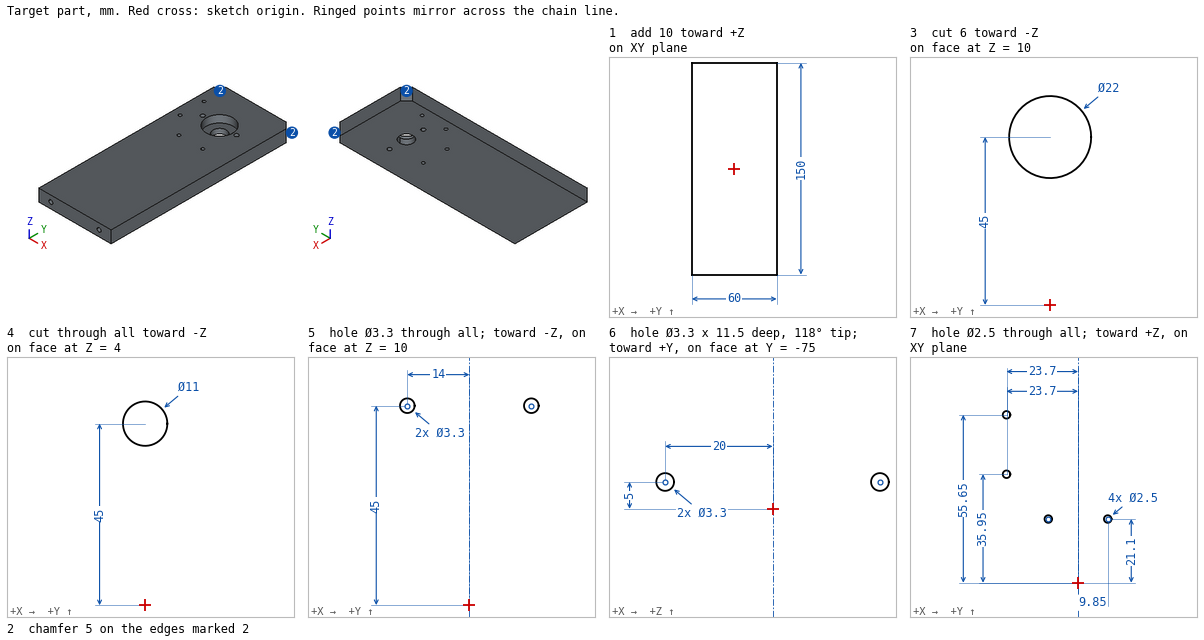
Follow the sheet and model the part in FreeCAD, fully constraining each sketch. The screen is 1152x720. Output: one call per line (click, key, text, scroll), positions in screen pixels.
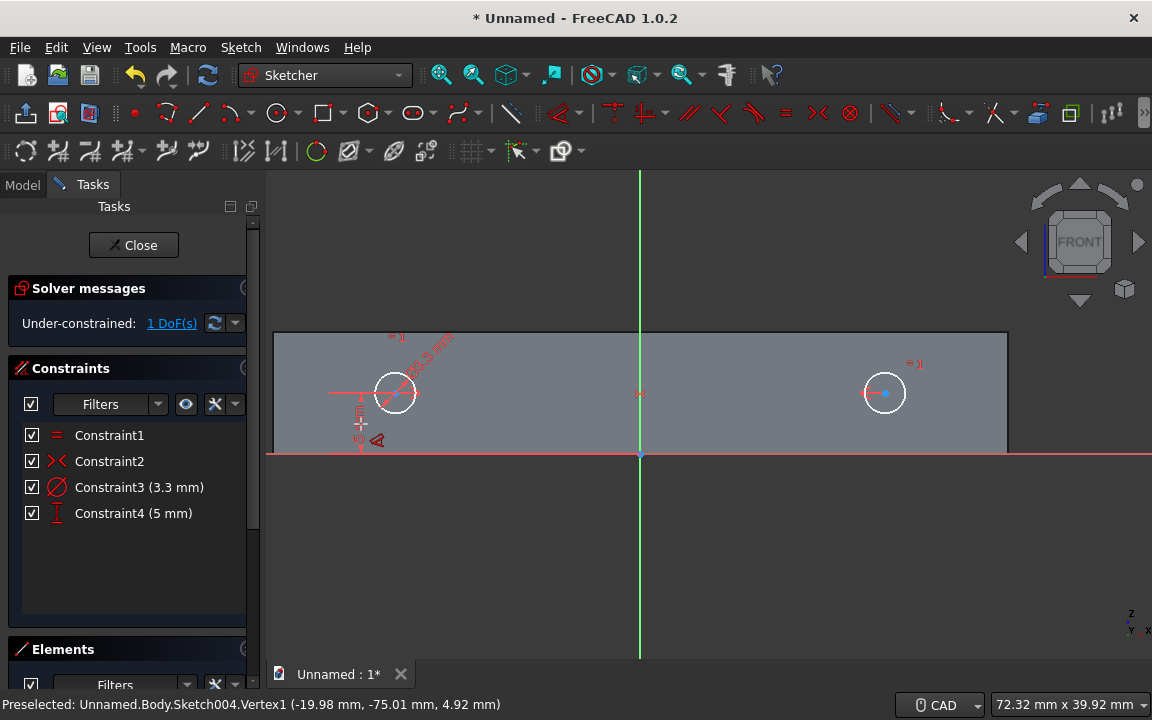
click(395, 393)
click(518, 488)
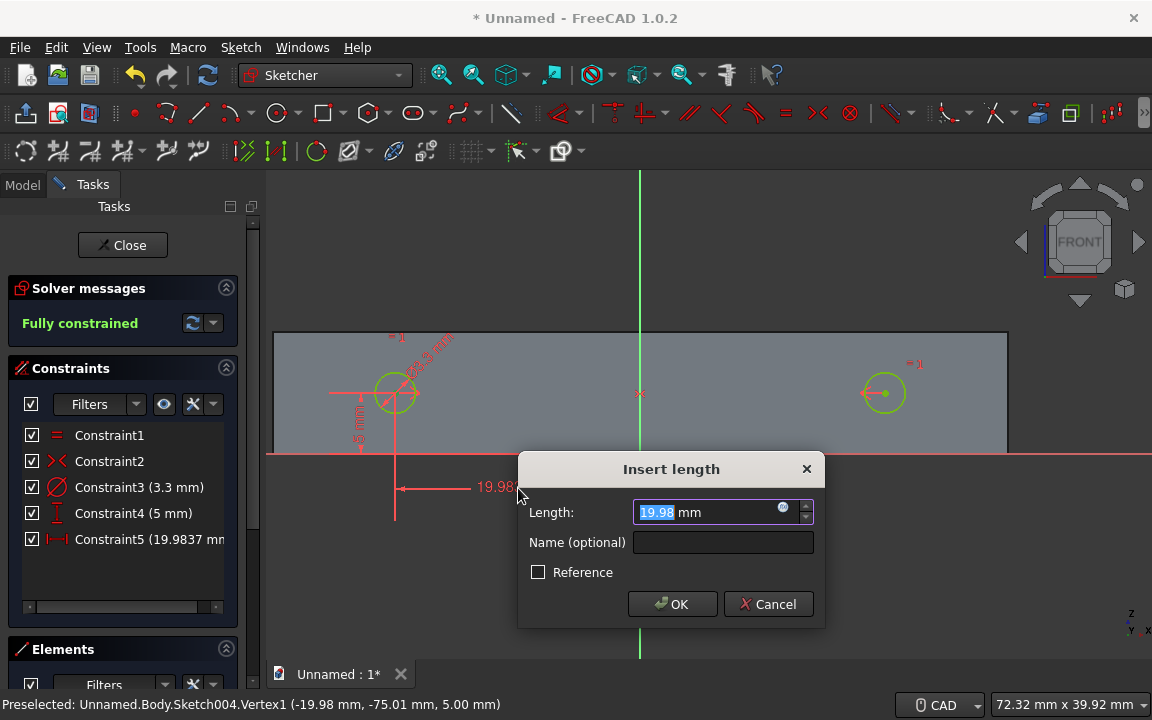
text(20)
key(Return)
key(Escape)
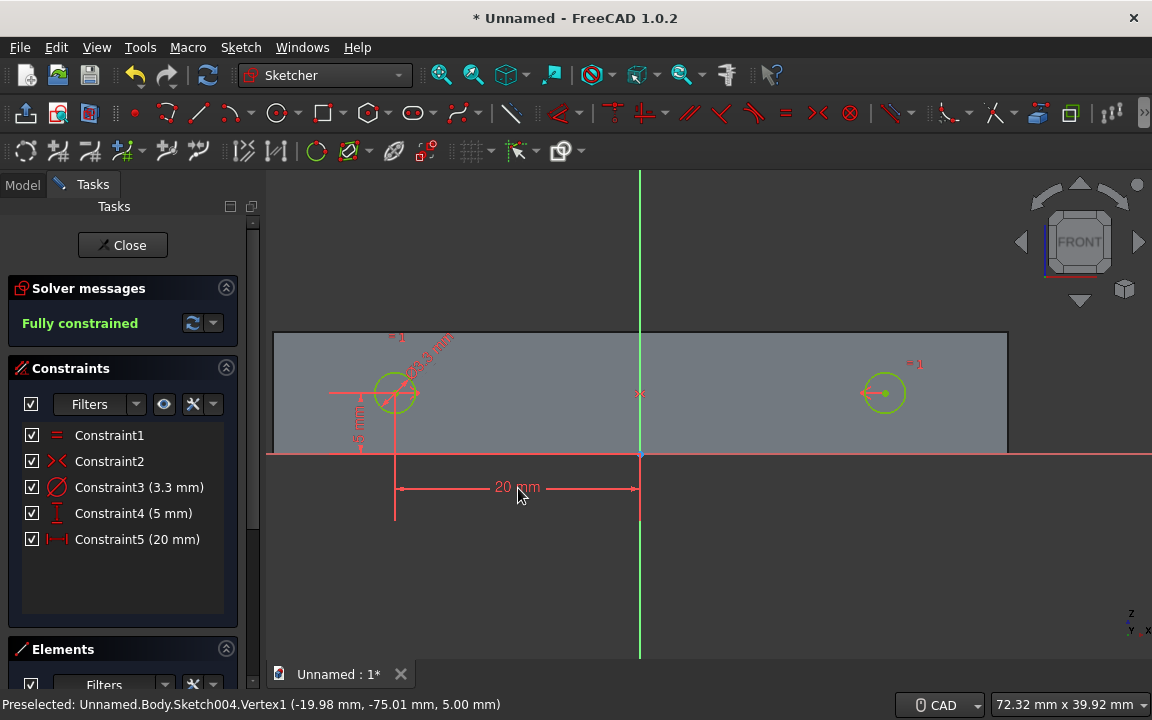
click(123, 245)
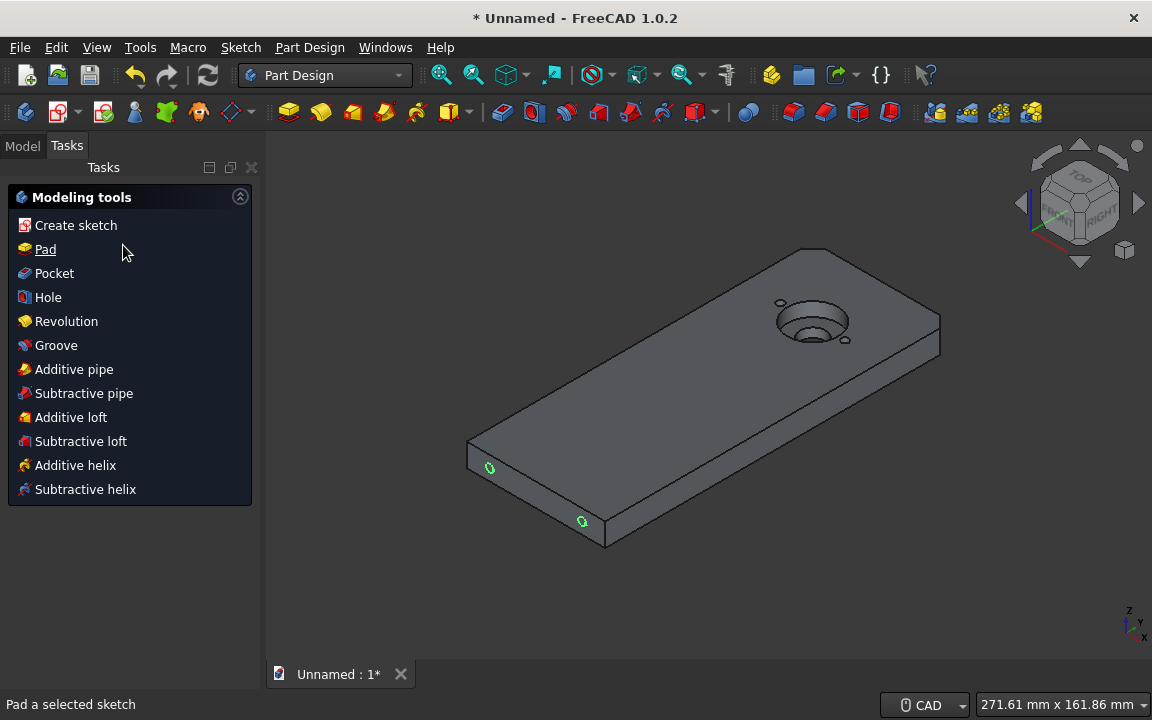
click(536, 112)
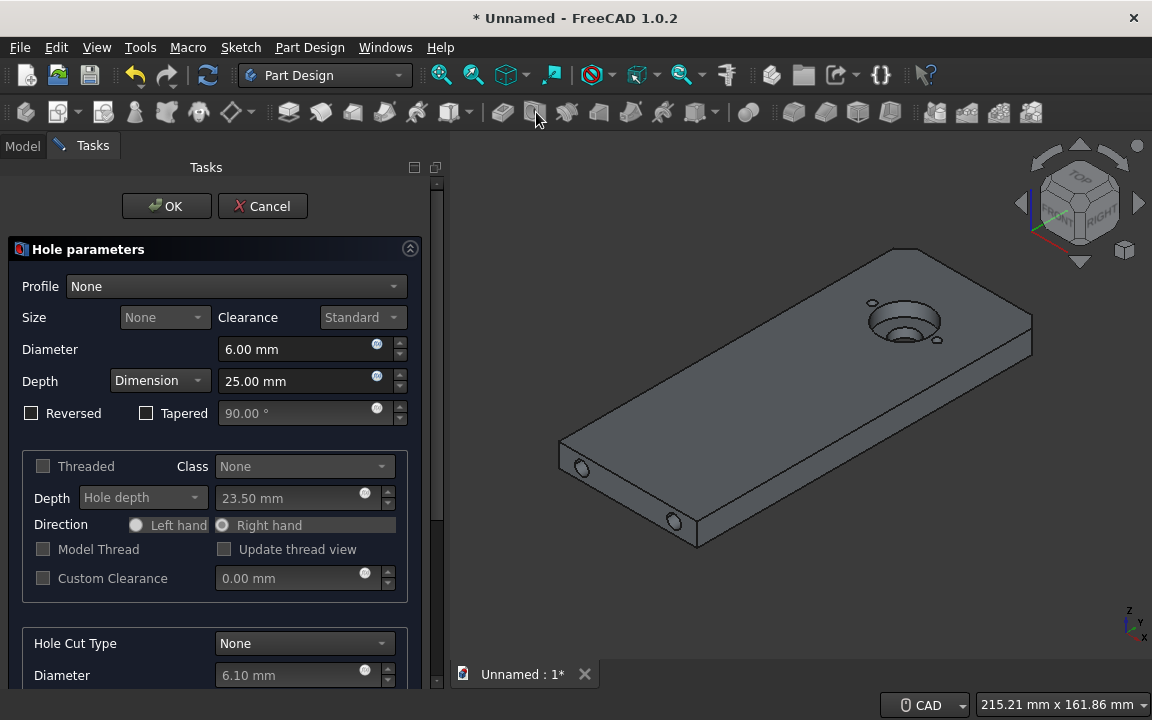
triple_click(305, 349)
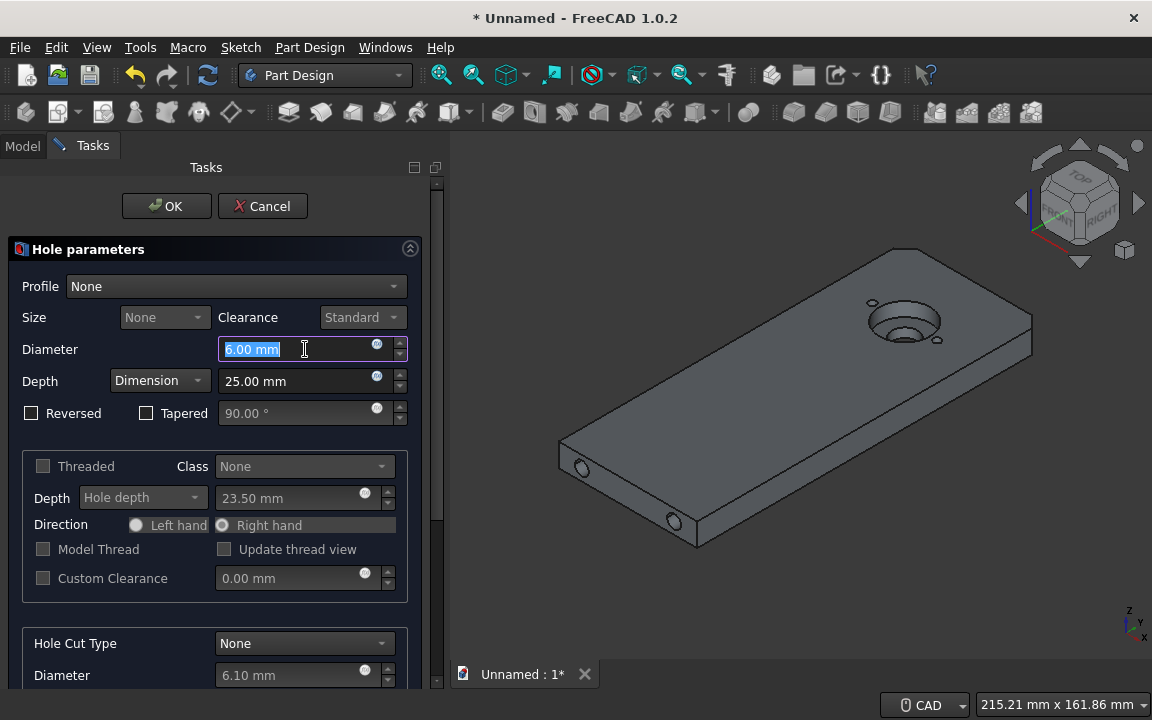
text(3.3)
key(Tab)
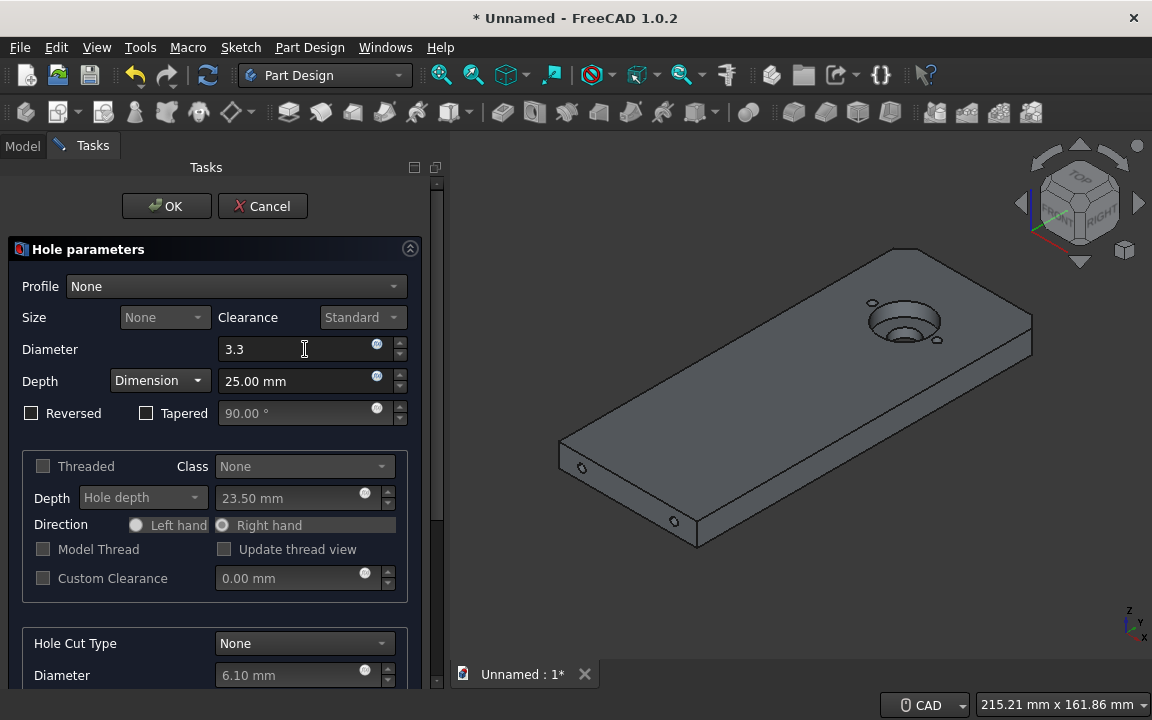
triple_click(305, 381)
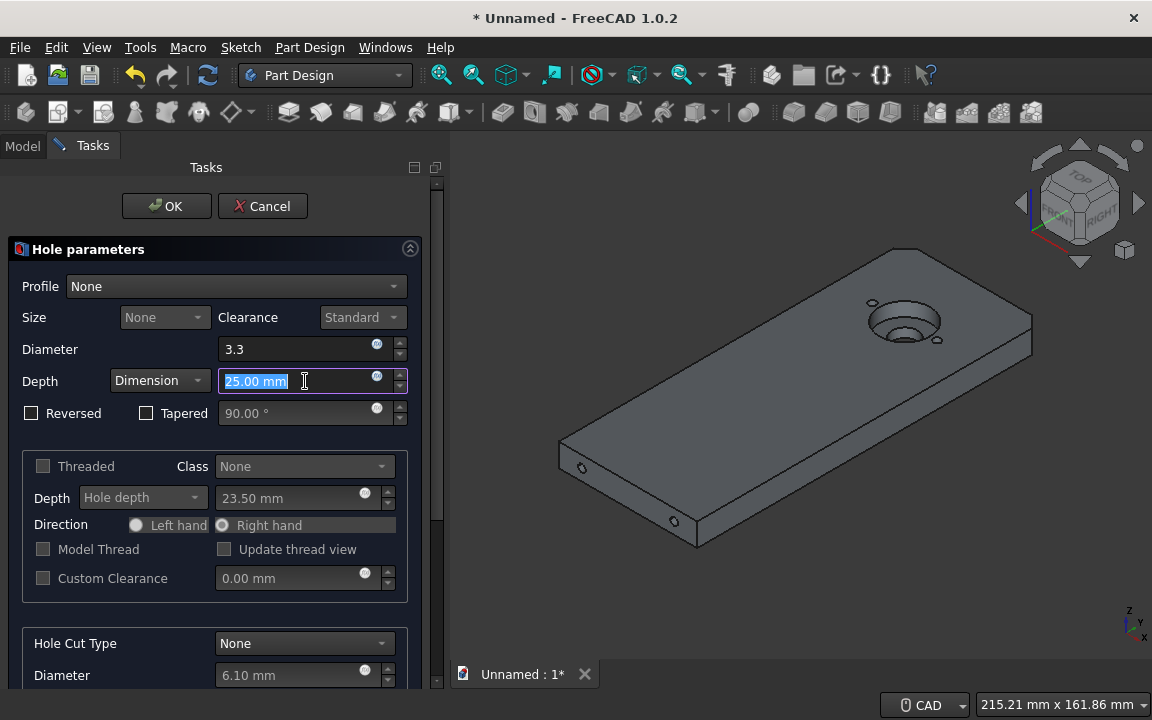
text(11.5)
key(Tab)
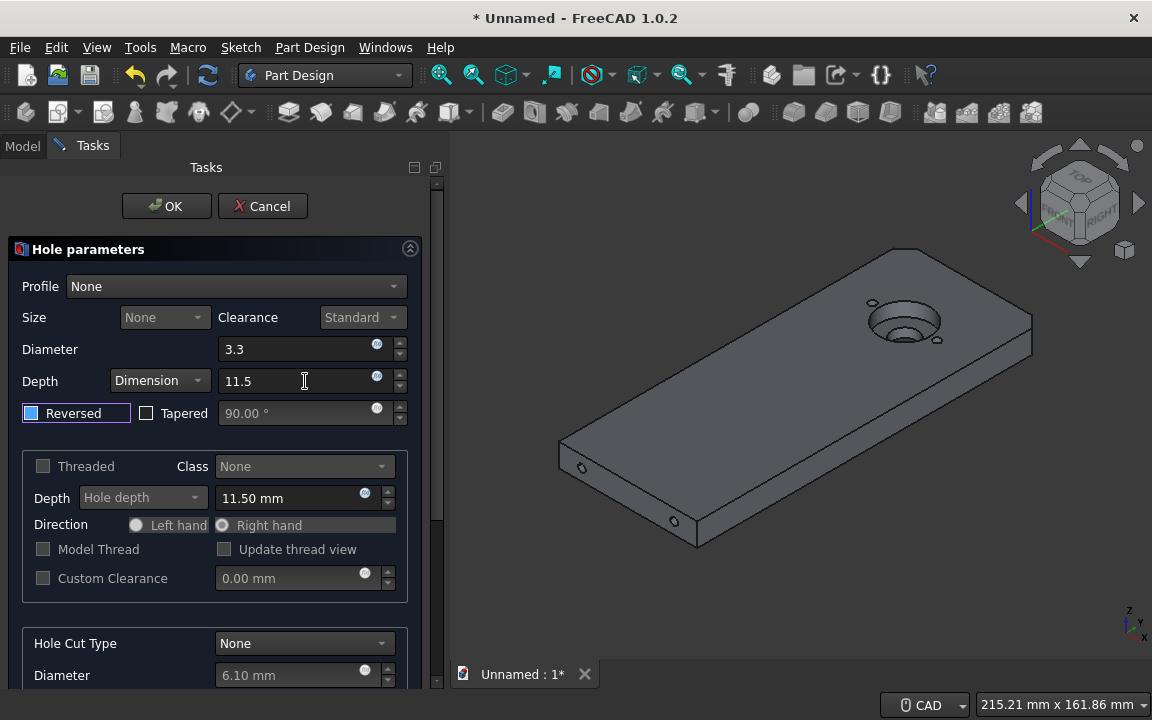
click(167, 206)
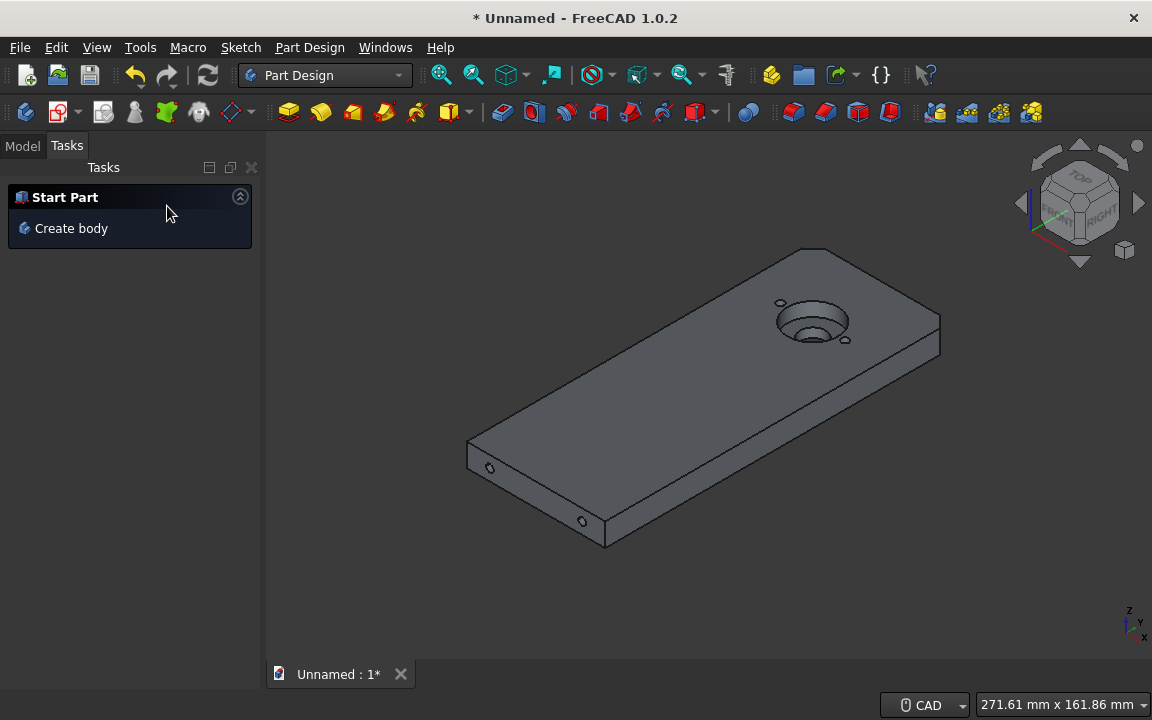
click(58, 112)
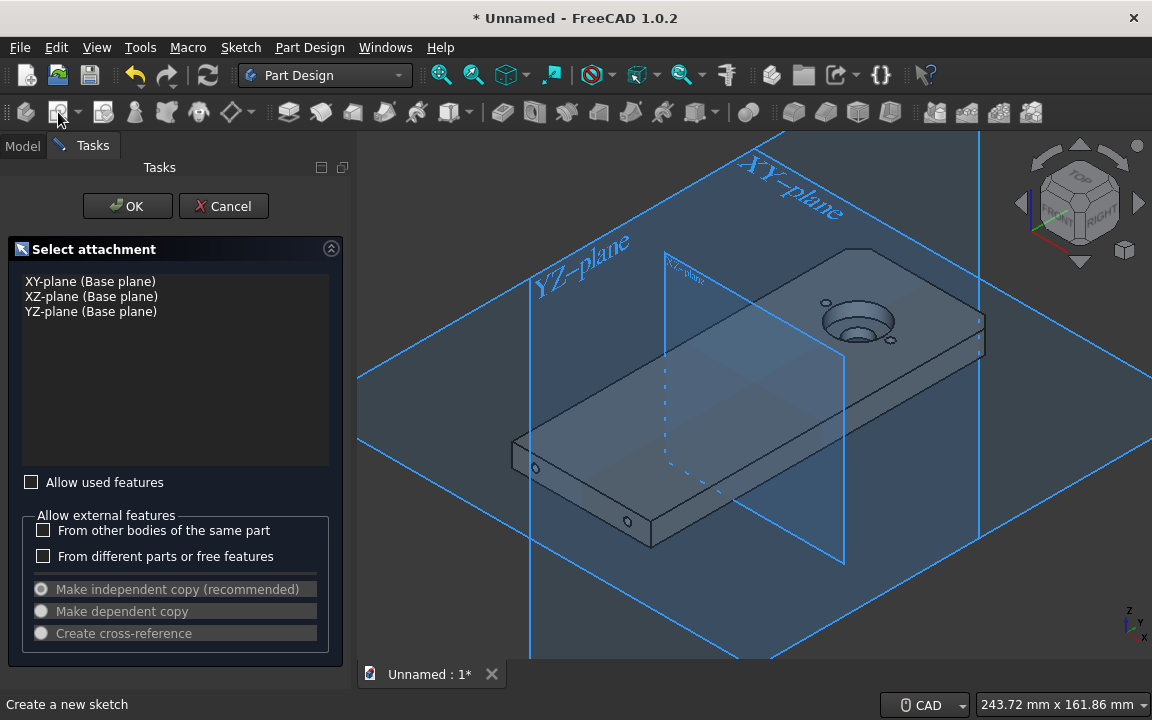
click(82, 282)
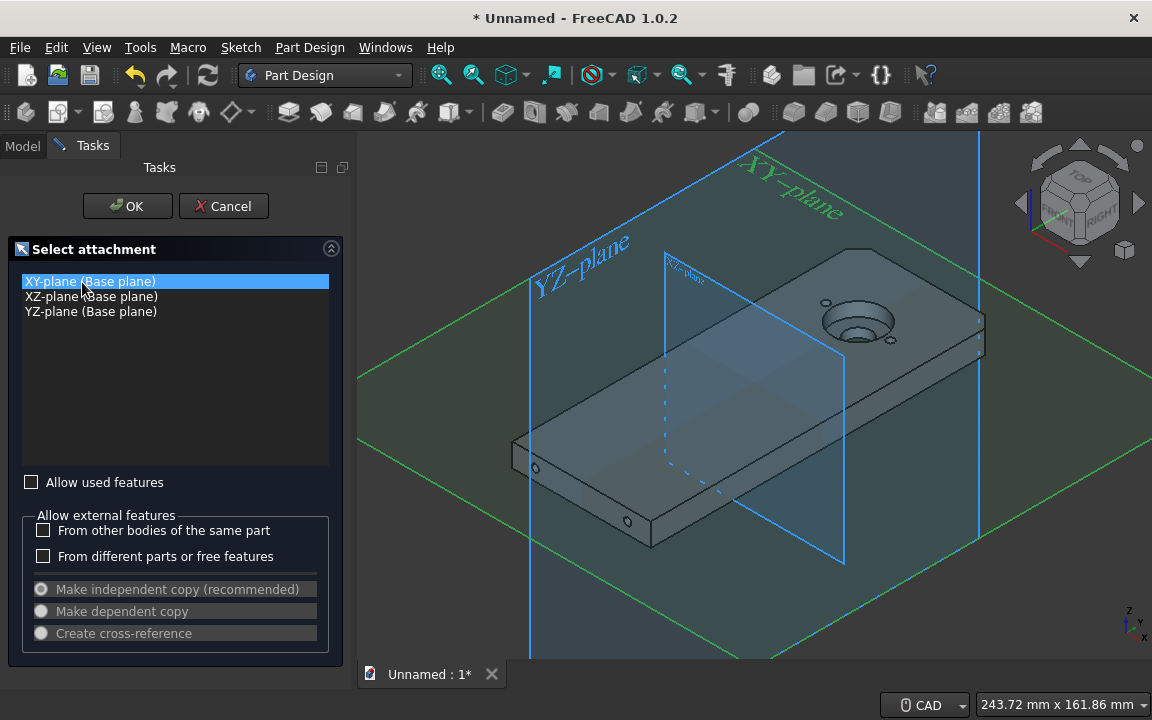
click(128, 206)